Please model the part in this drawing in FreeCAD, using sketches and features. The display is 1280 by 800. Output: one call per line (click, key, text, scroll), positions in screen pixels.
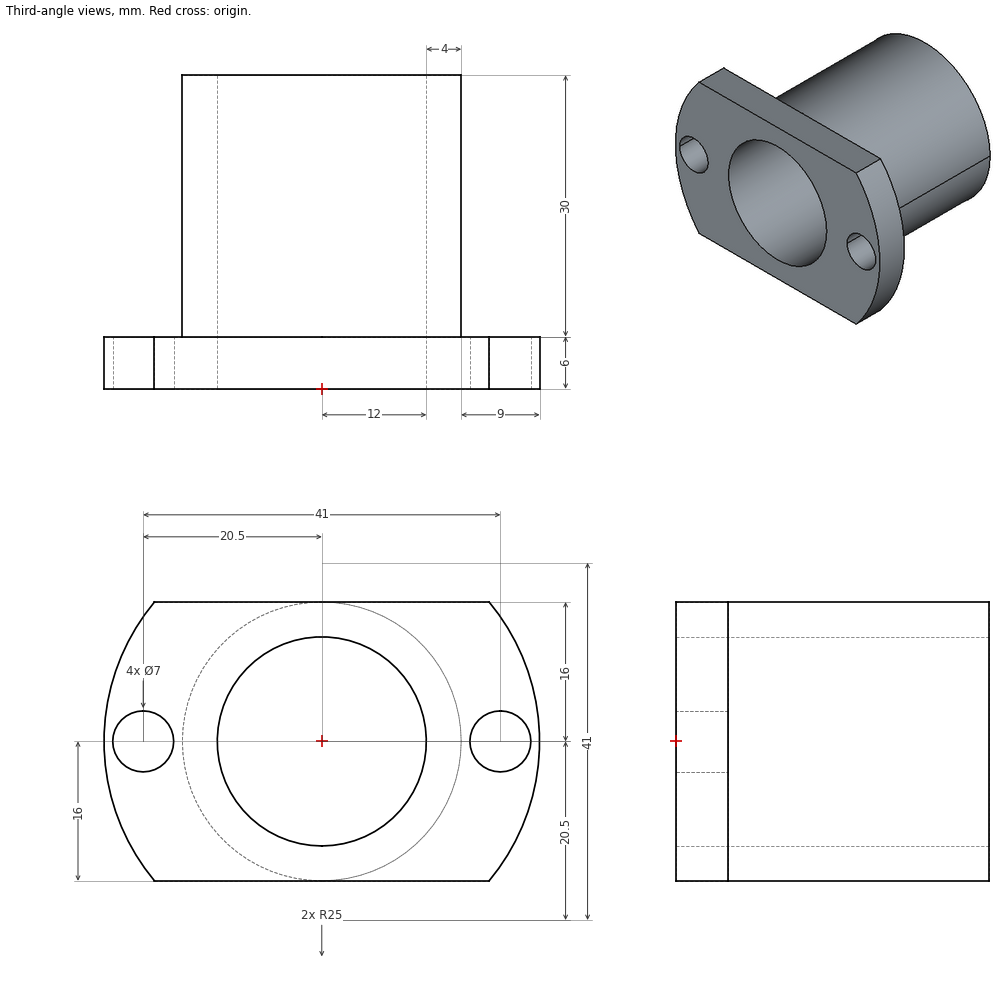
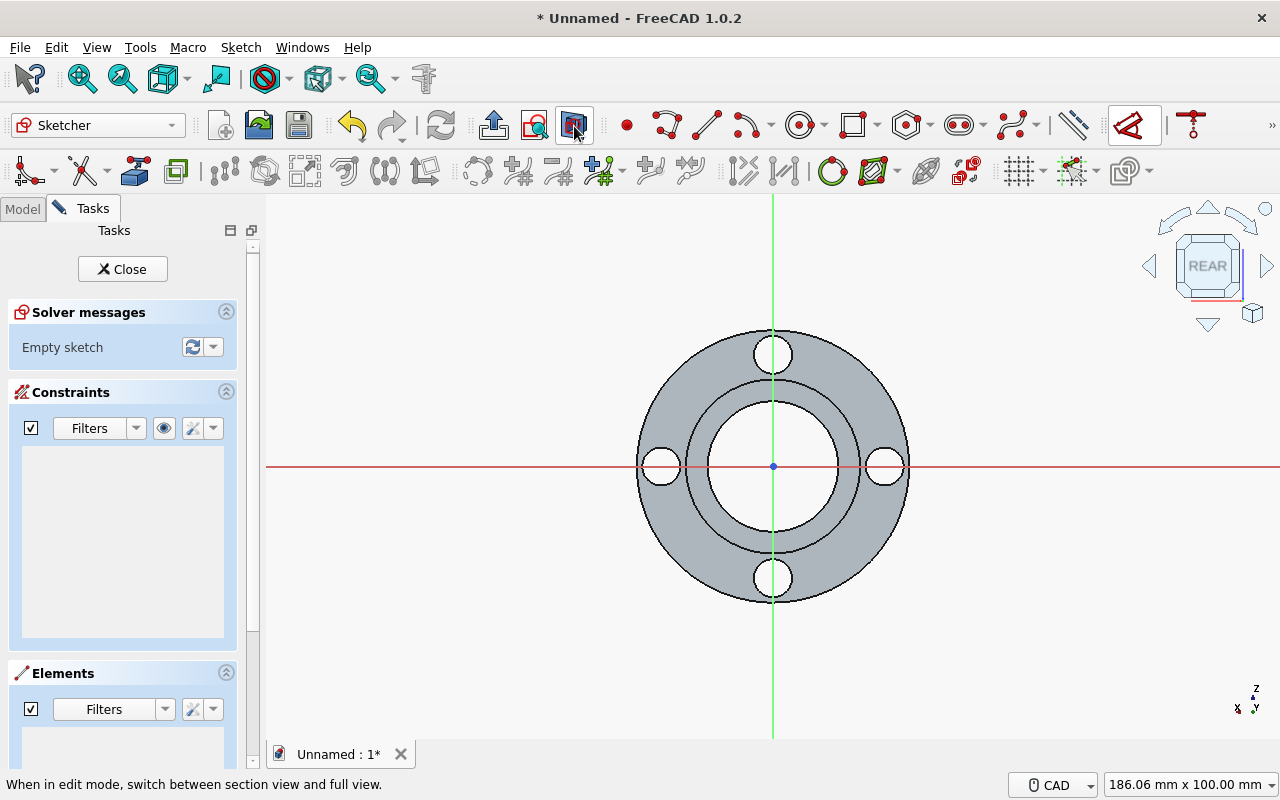
click(708, 126)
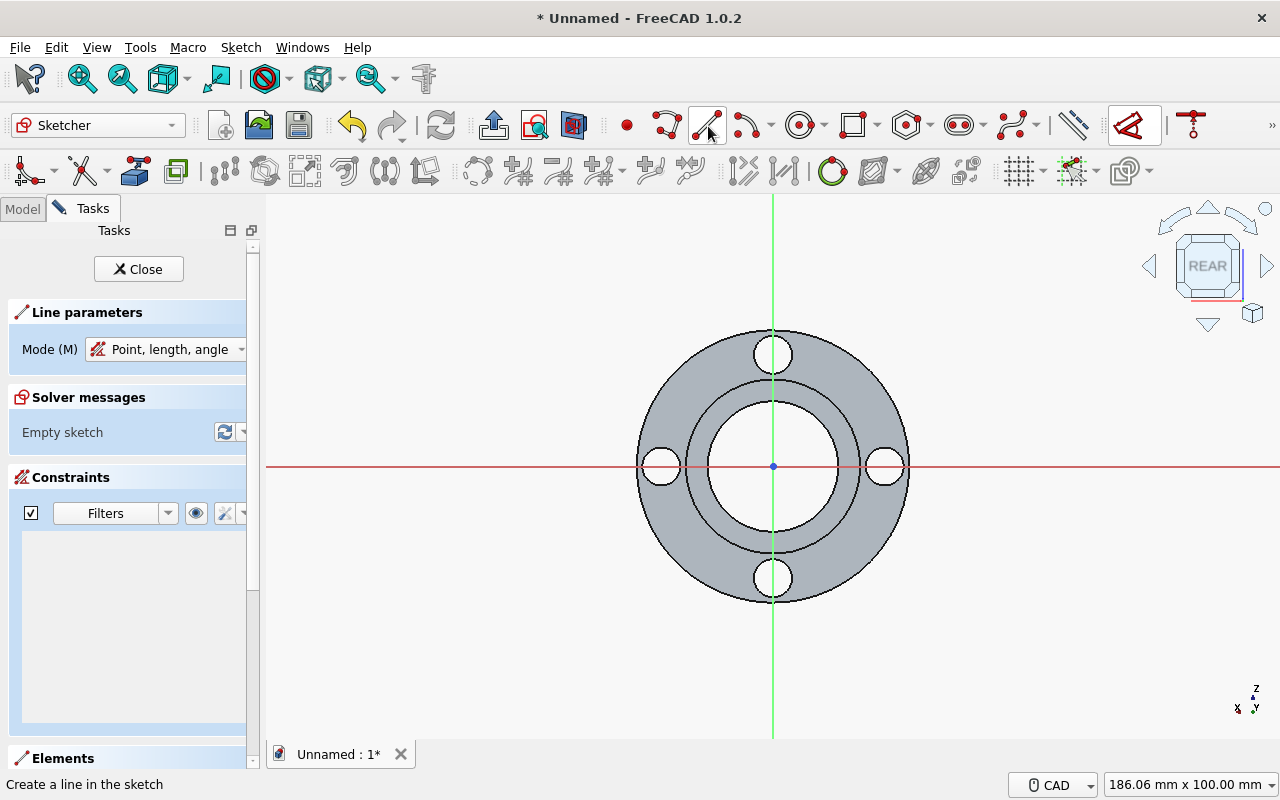
click(878, 554)
click(668, 554)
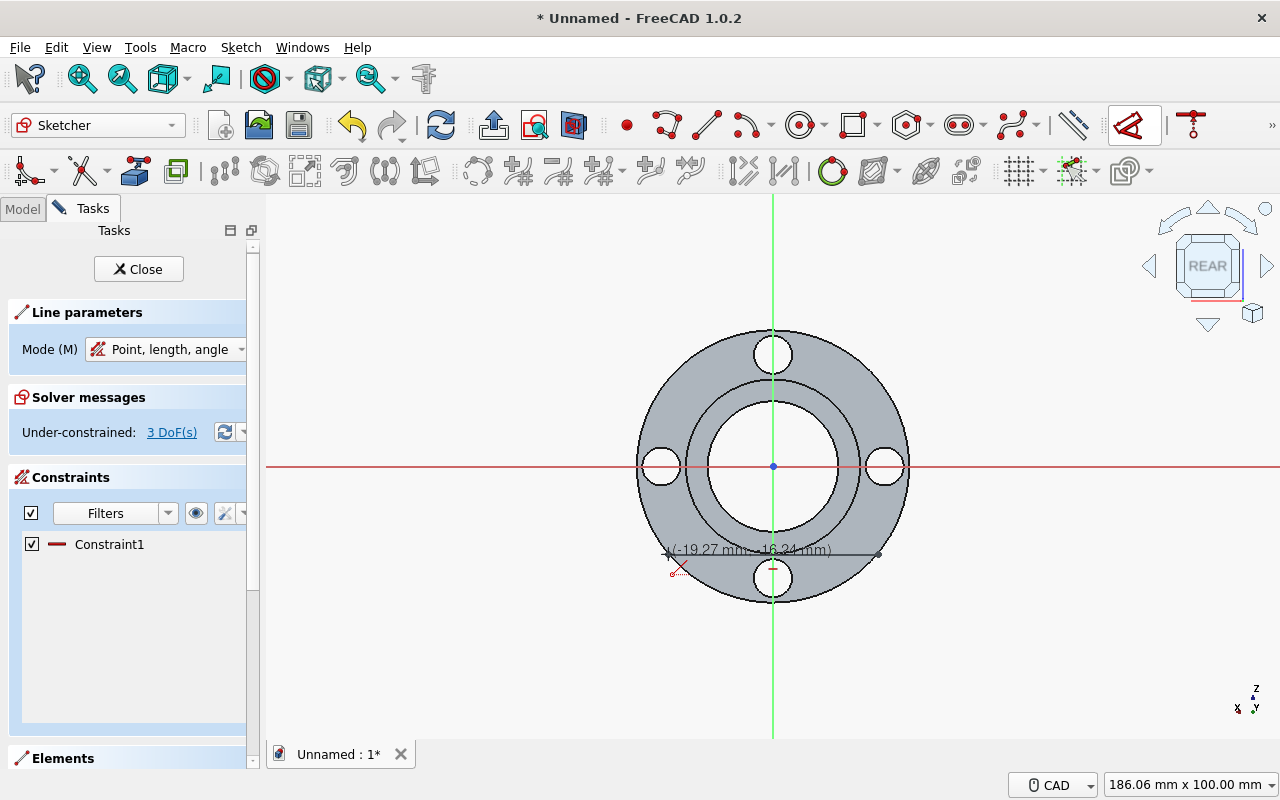
click(774, 126)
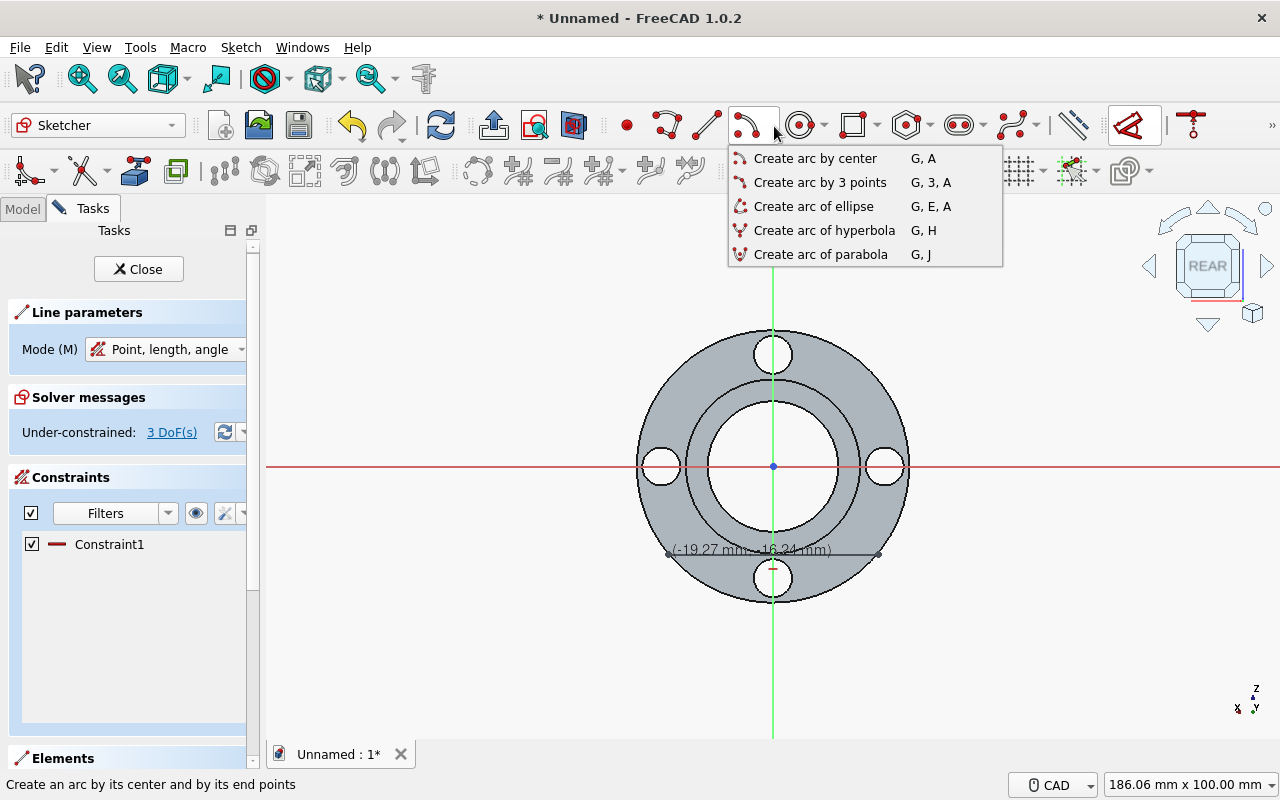
click(866, 182)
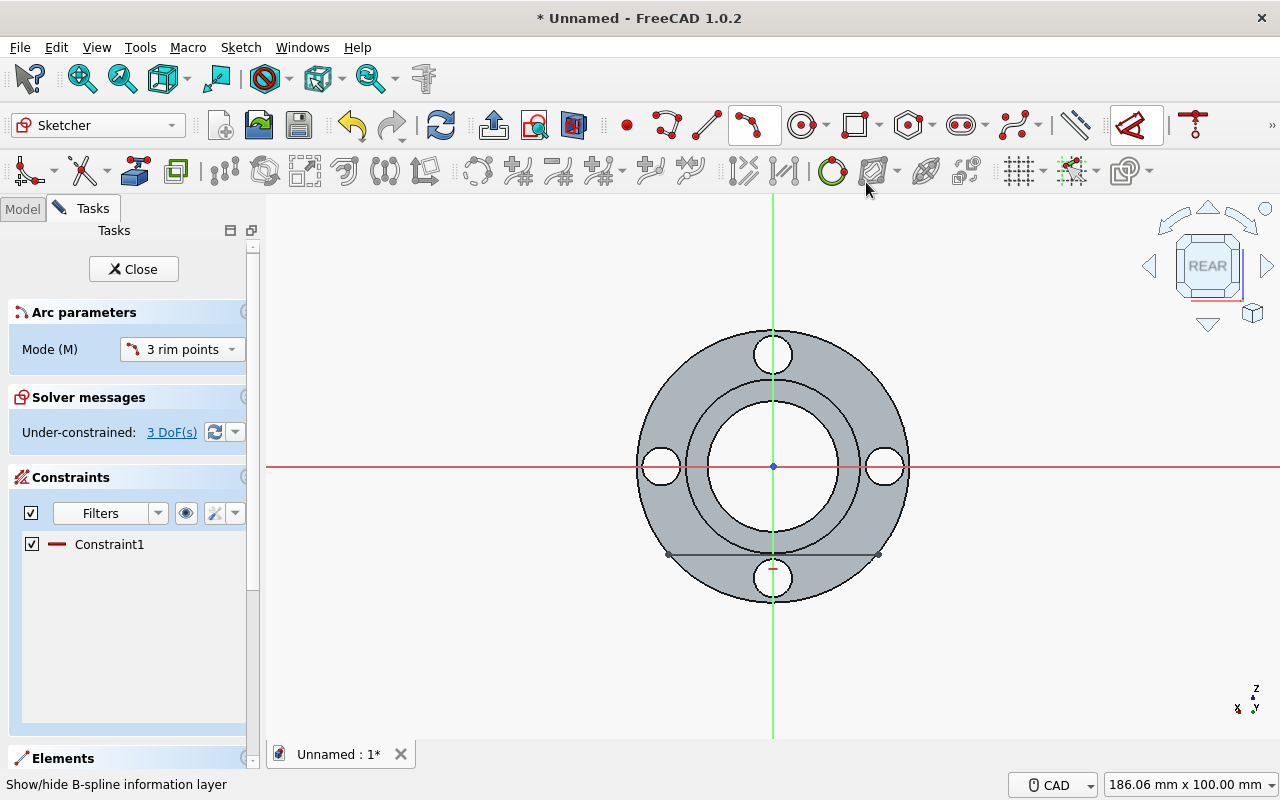
click(668, 555)
click(878, 555)
click(749, 601)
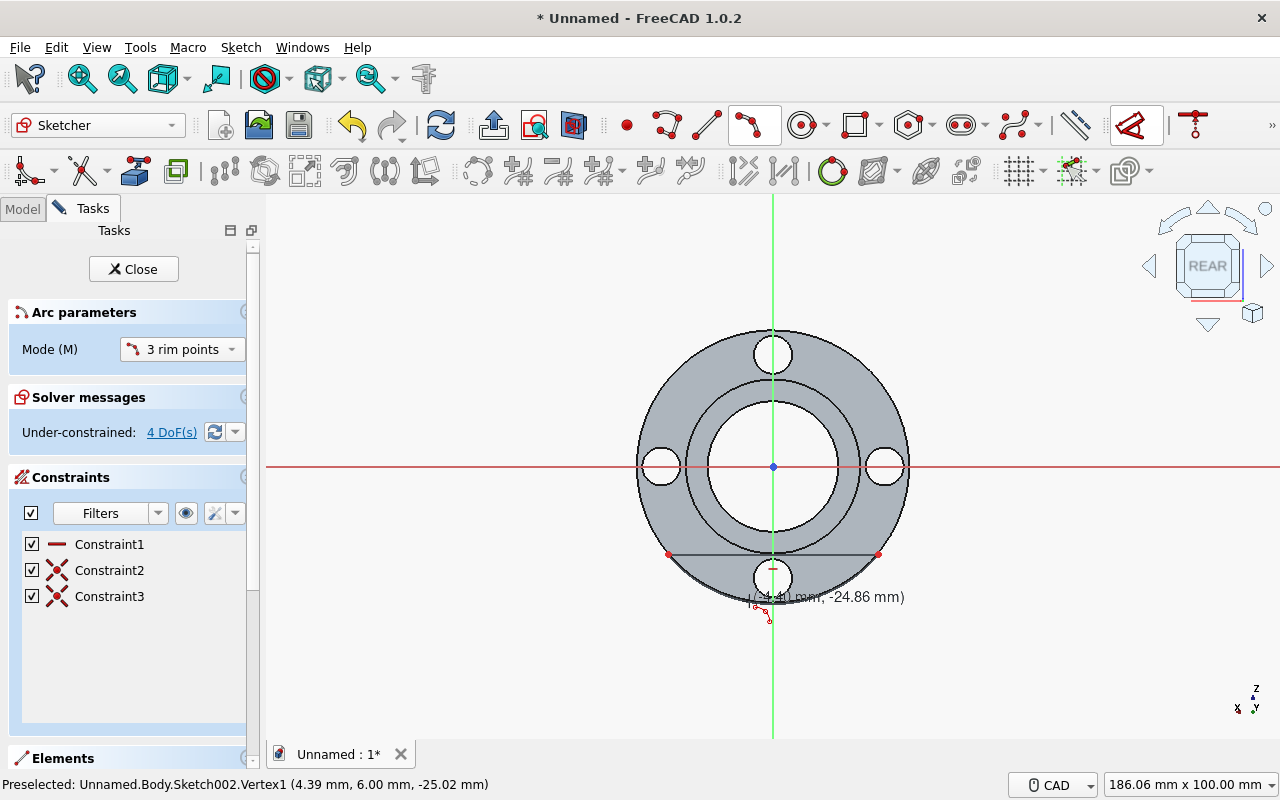
click(708, 126)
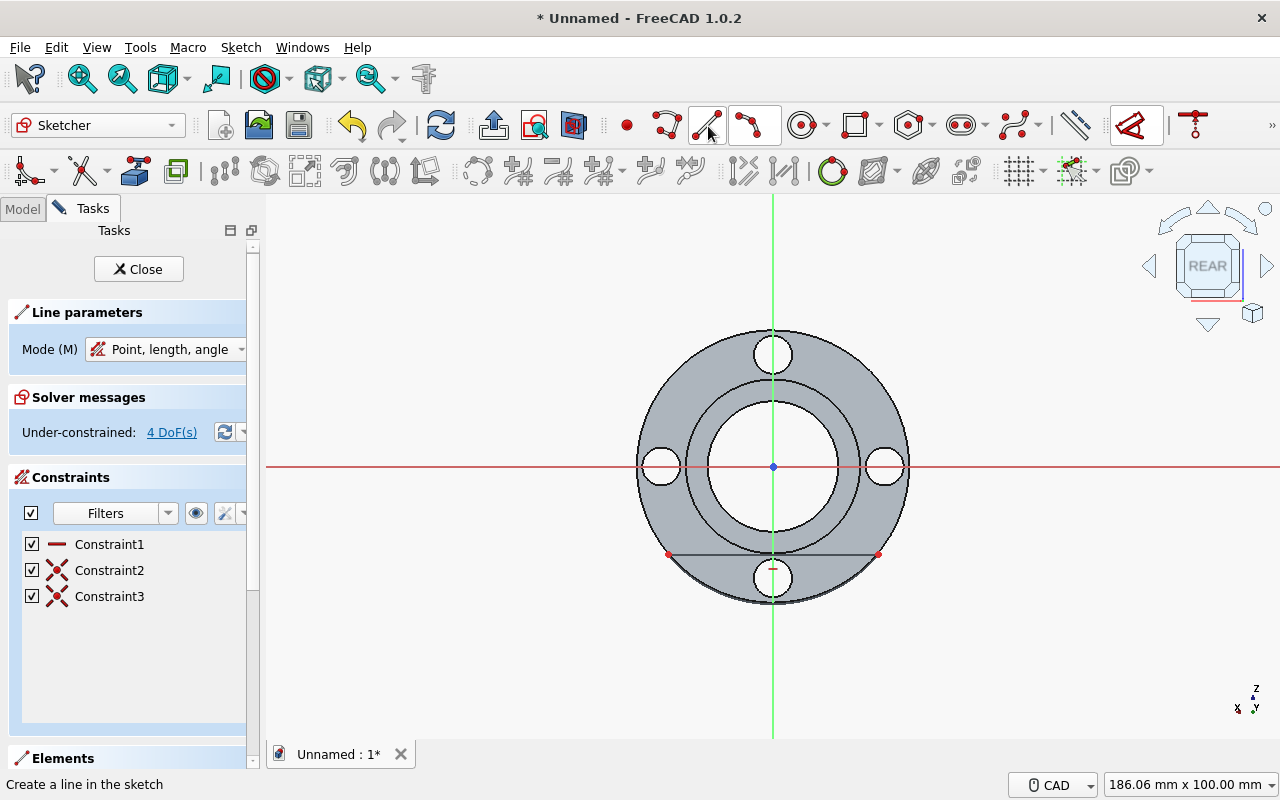
click(668, 379)
click(878, 379)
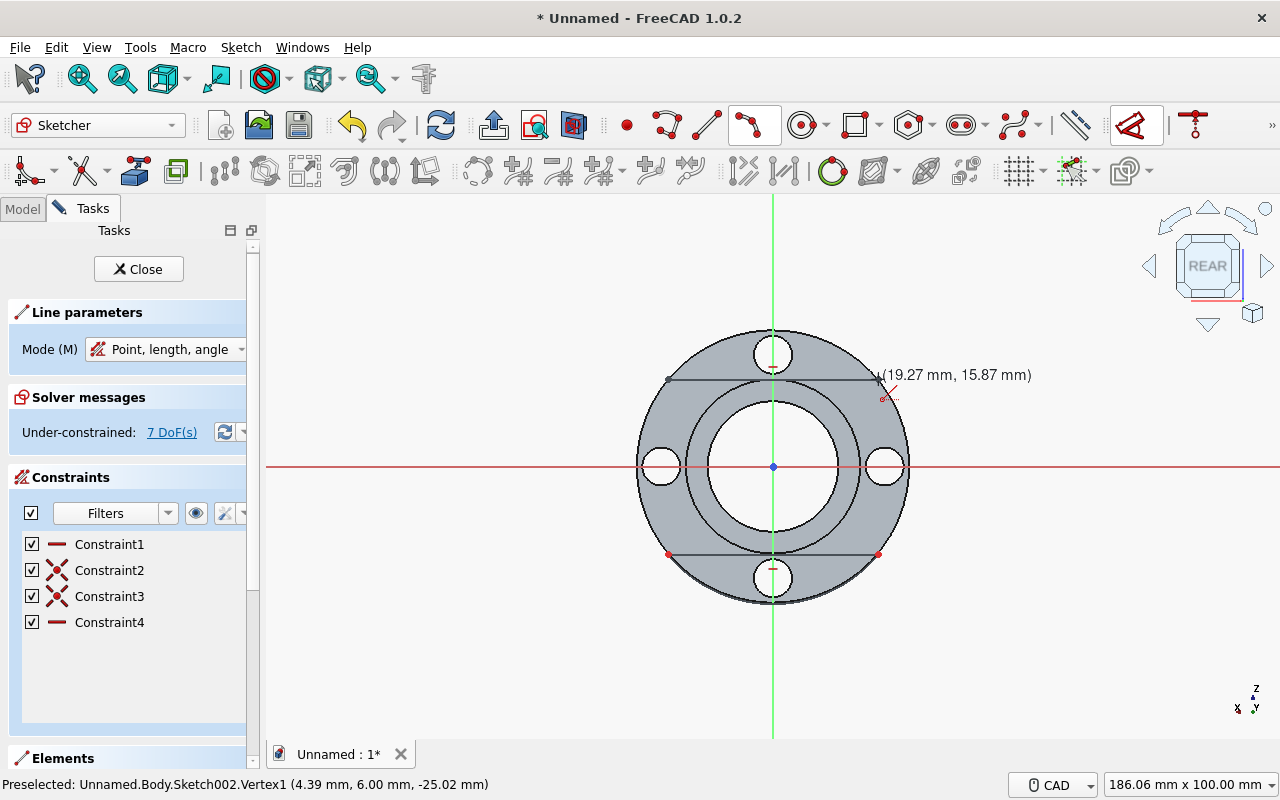
click(748, 126)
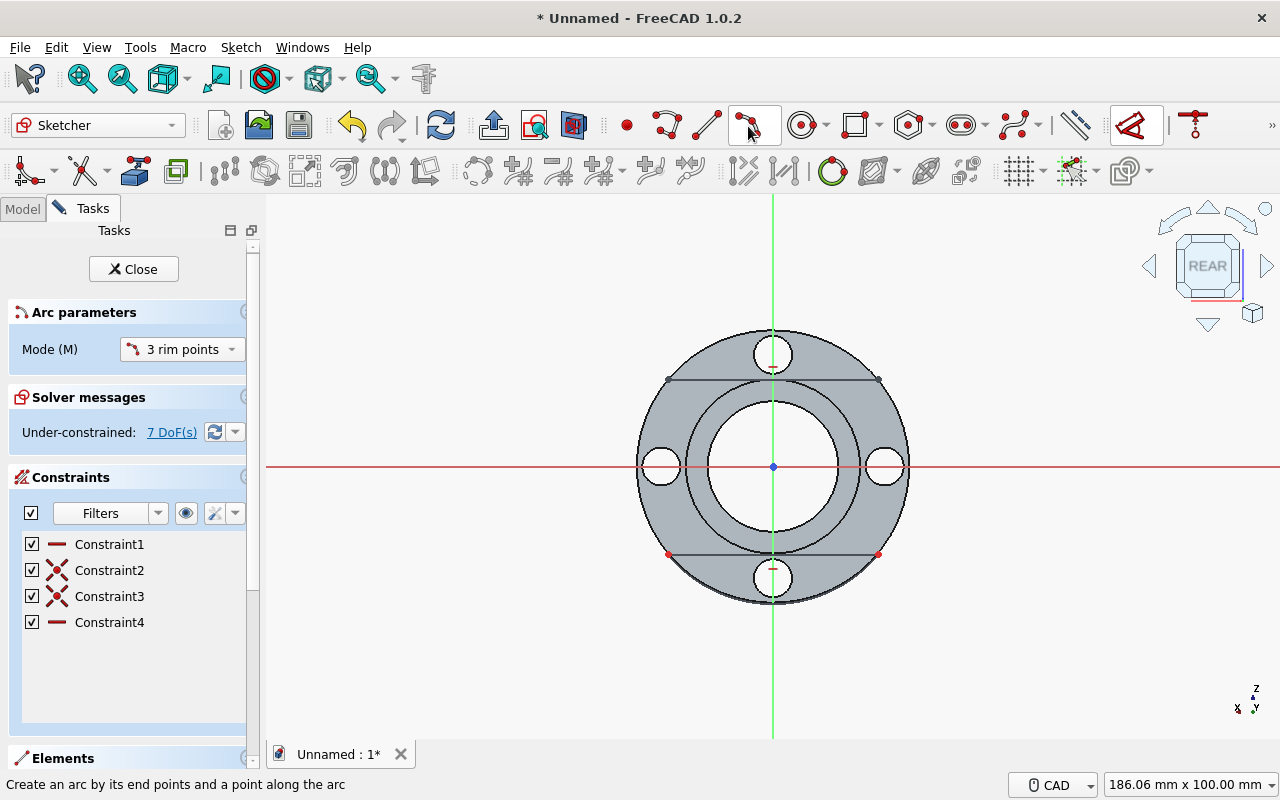
click(878, 380)
click(668, 380)
click(797, 332)
key(Escape)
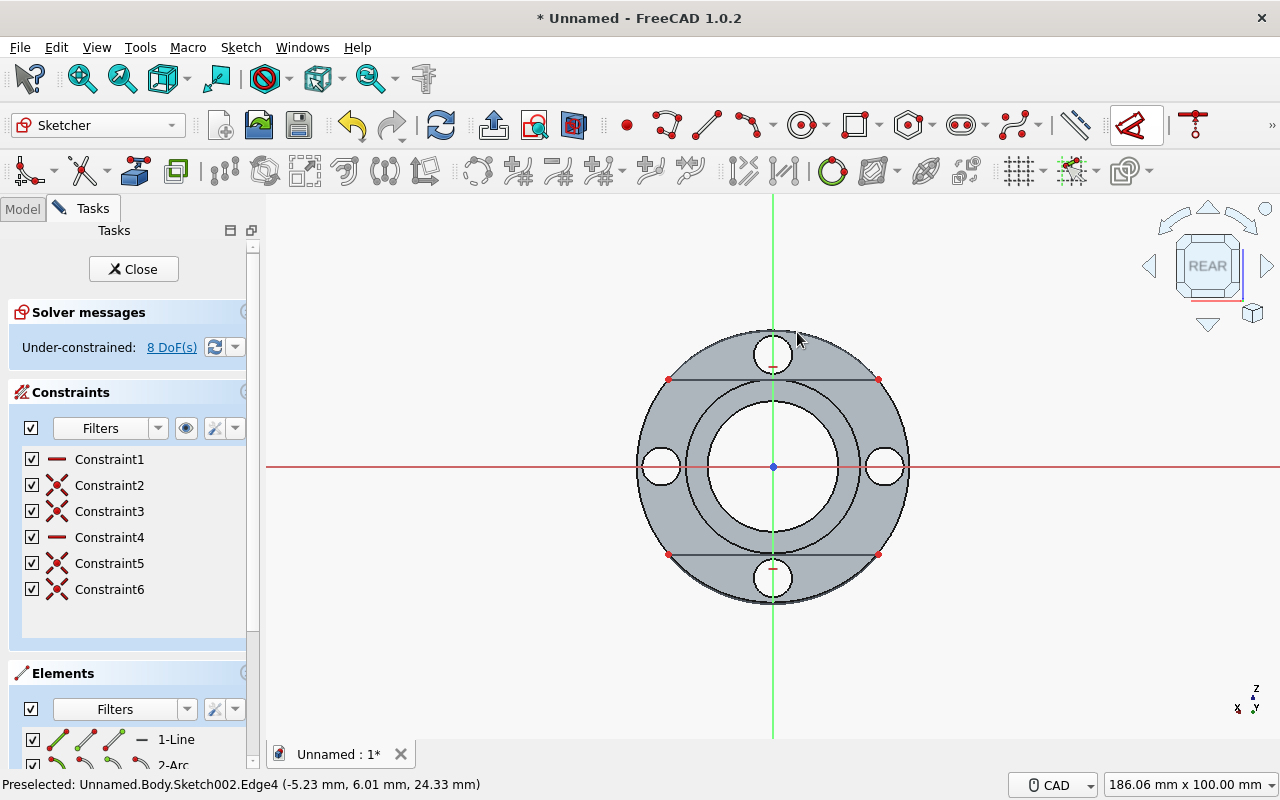
click(726, 596)